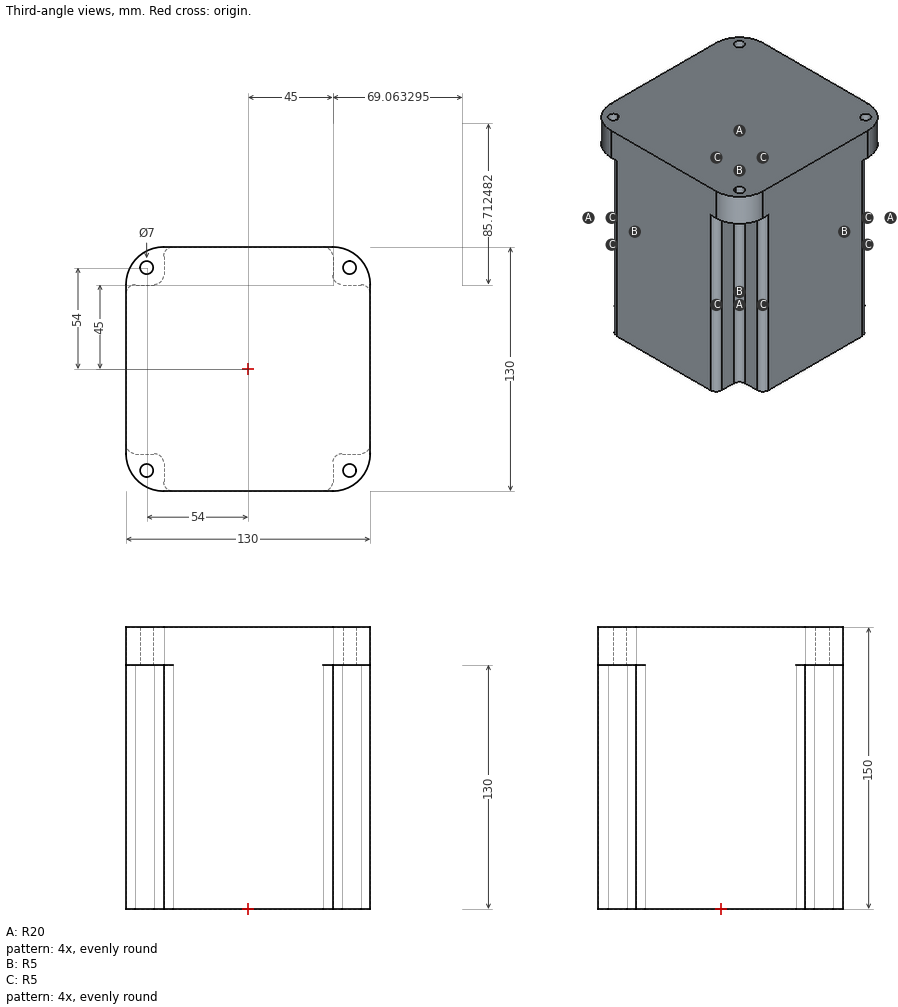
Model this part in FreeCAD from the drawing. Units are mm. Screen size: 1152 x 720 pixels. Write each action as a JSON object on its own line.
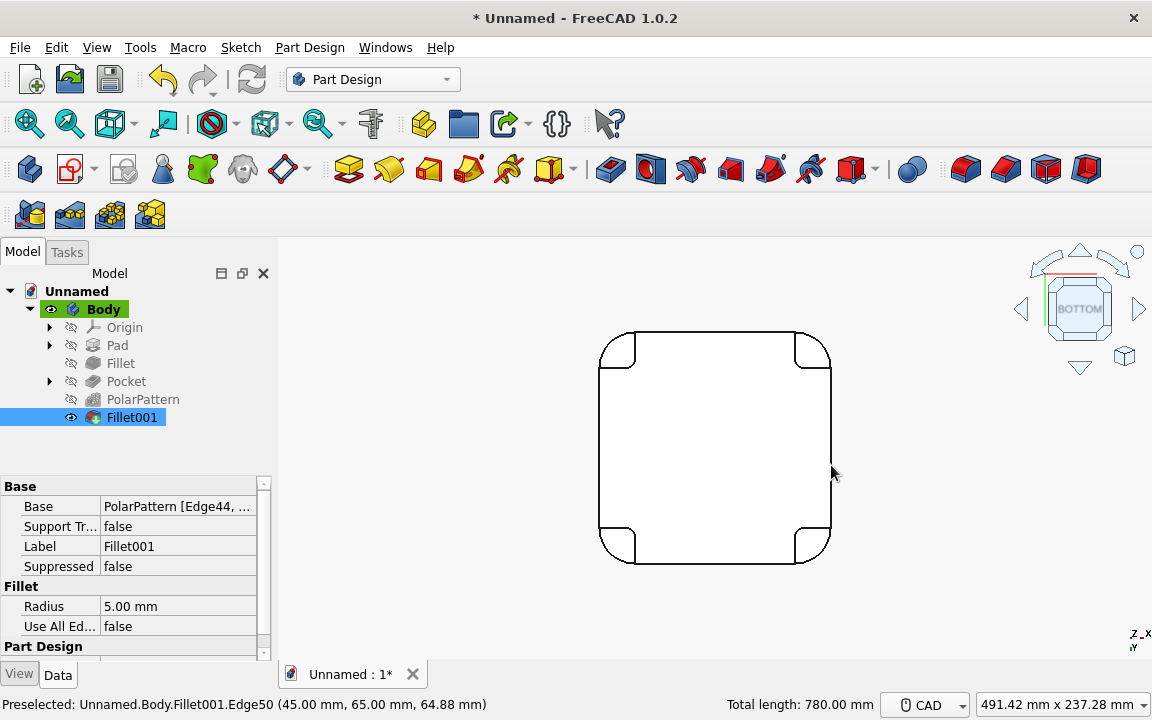
{"action": "key", "text": "4"}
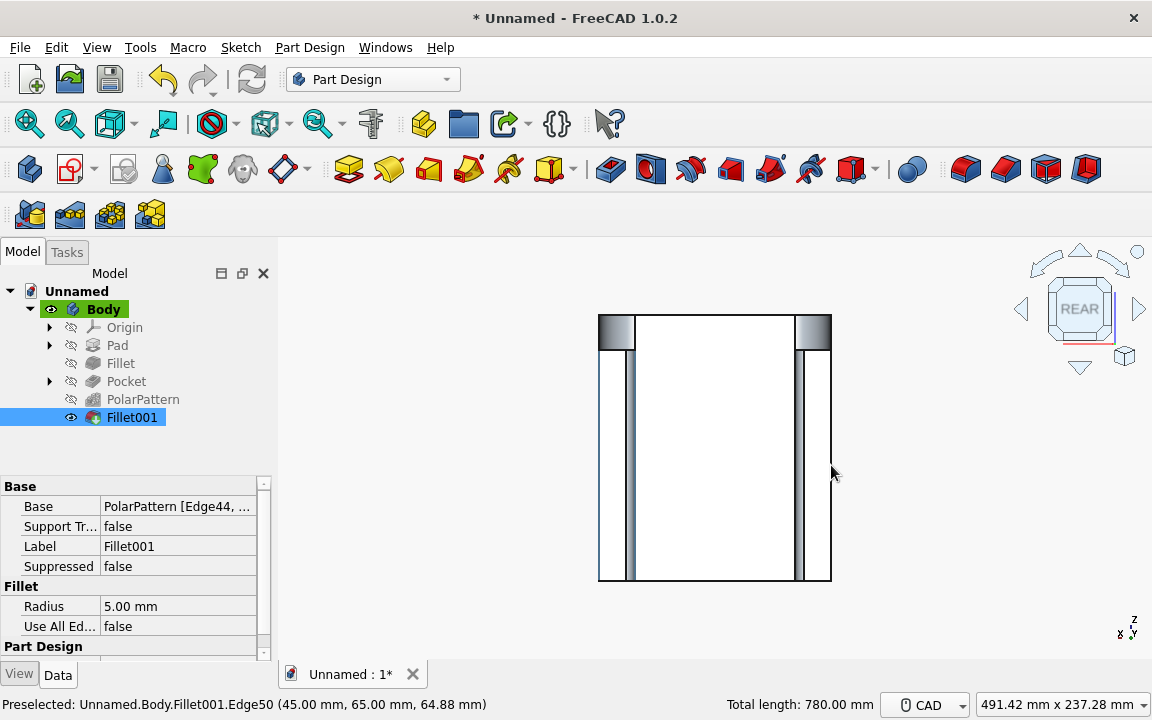
{"action": "left_click", "coordinate": [795, 465], "text": "ctrl"}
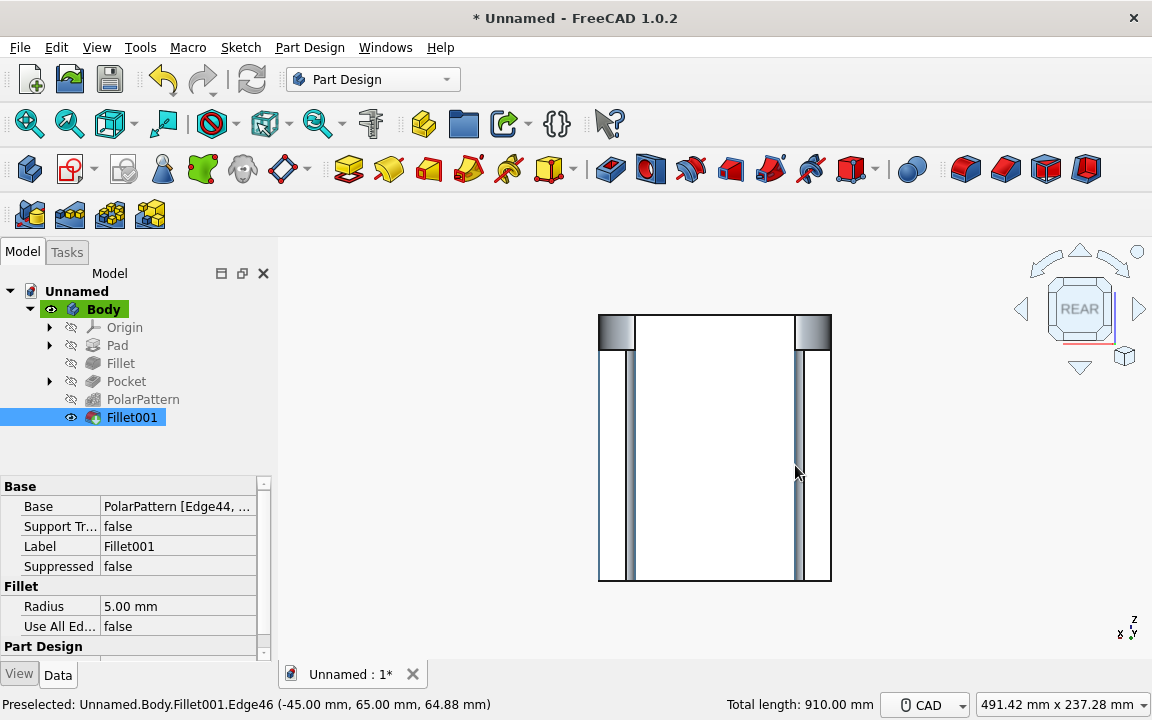
{"action": "left_click", "coordinate": [831, 465], "text": "ctrl"}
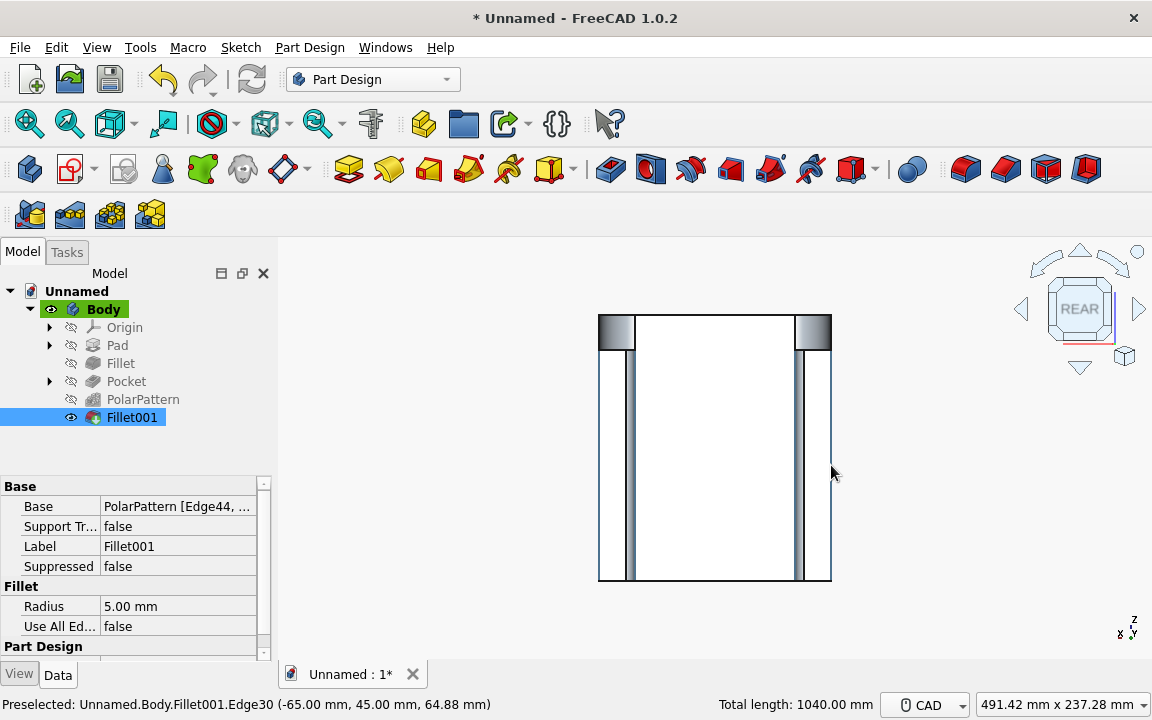
{"action": "left_click", "coordinate": [966, 170]}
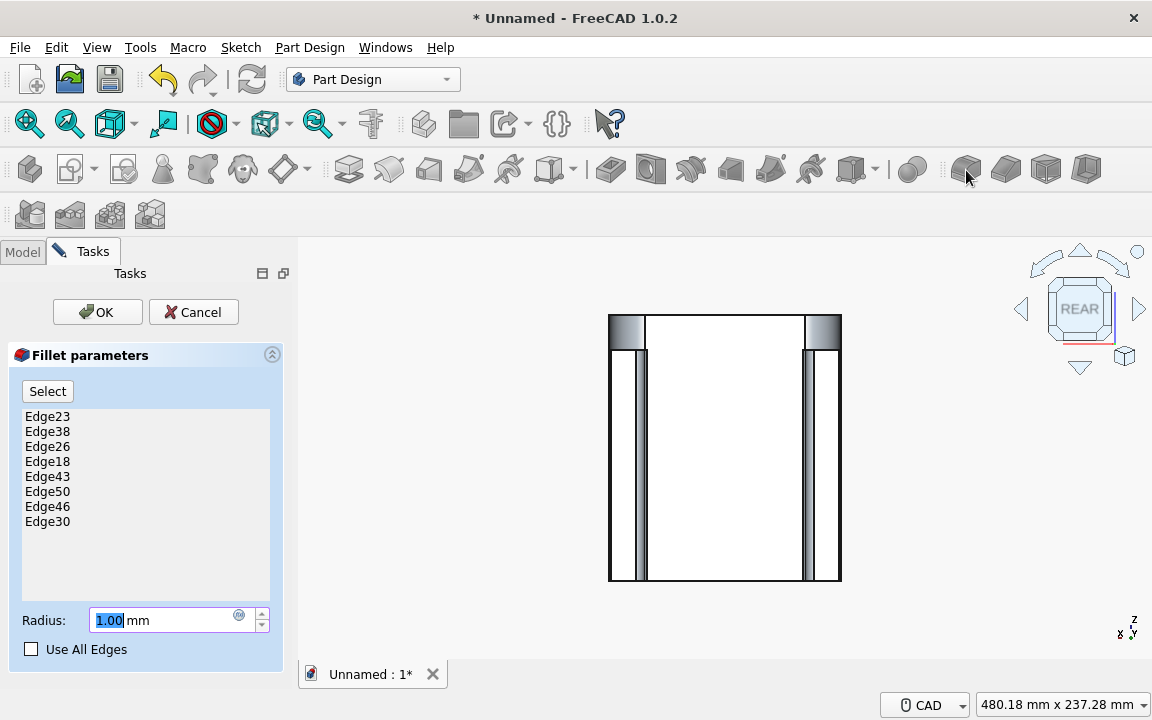
{"action": "type", "text": "5"}
{"action": "key", "text": "Tab"}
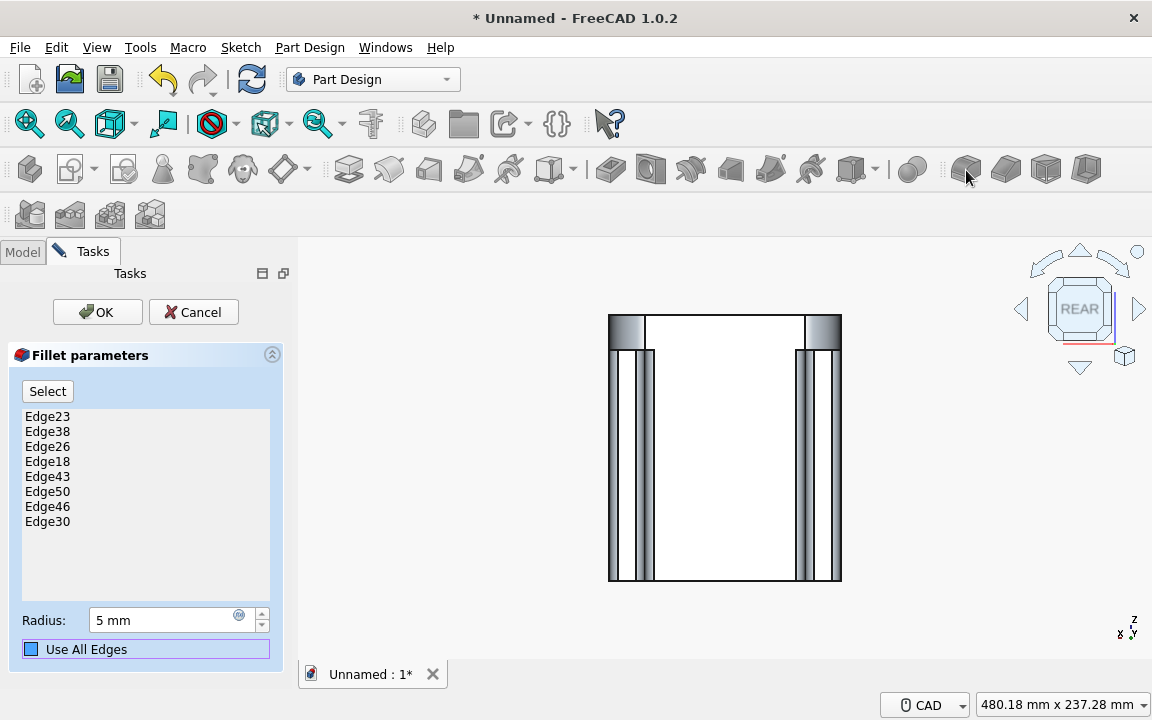
{"action": "left_click", "coordinate": [98, 312]}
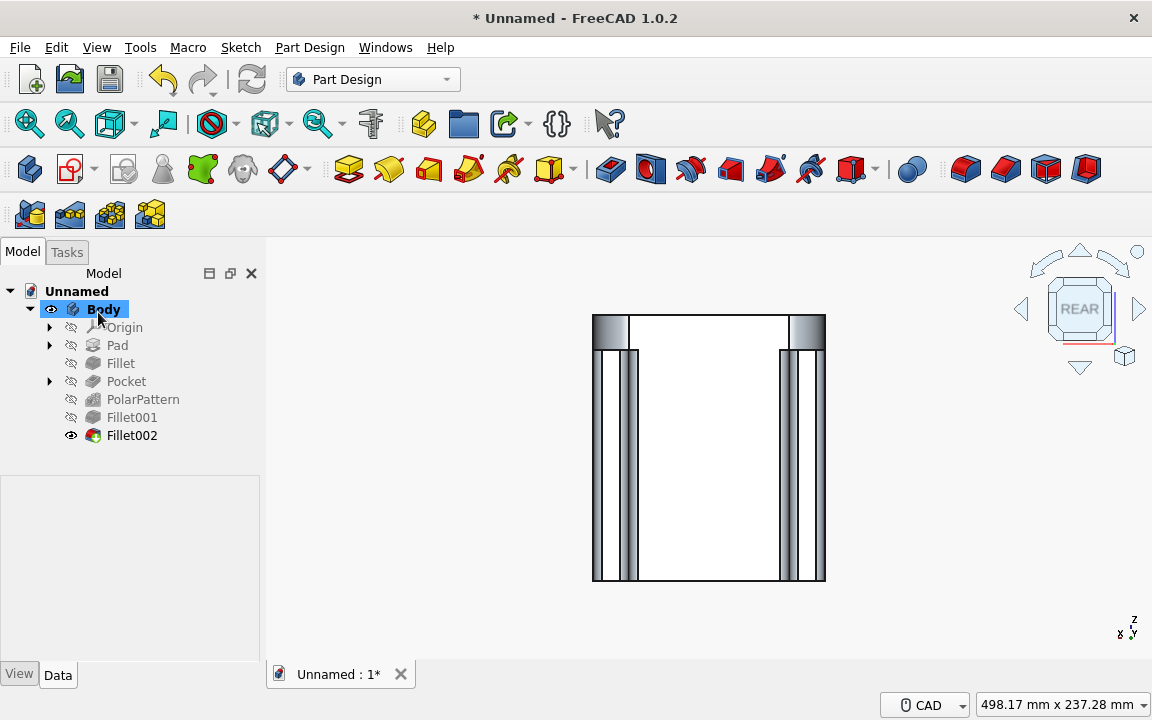
{"action": "key", "text": "5"}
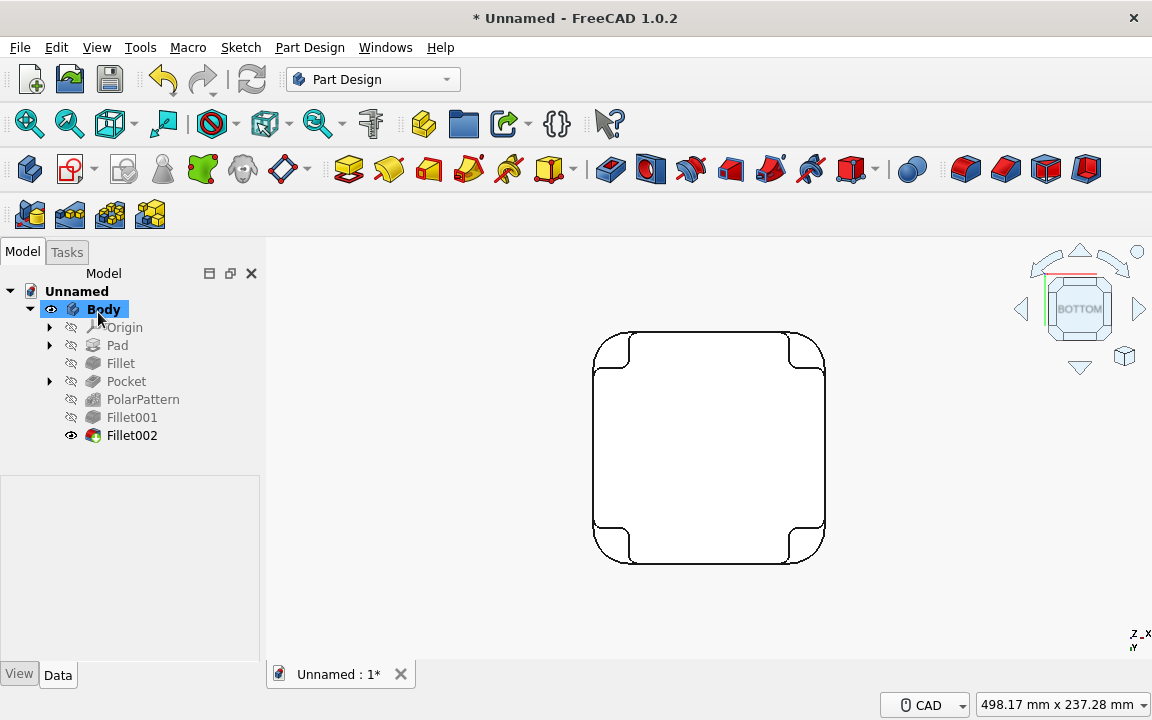
{"action": "left_click", "coordinate": [802, 354]}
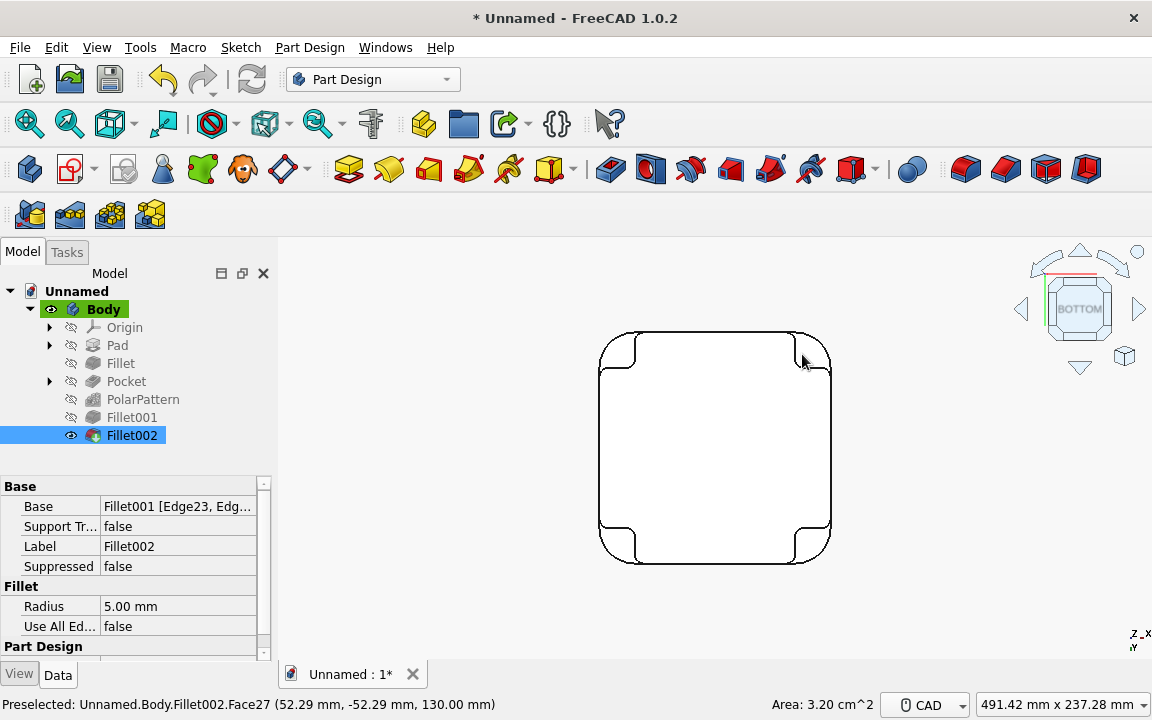
{"action": "left_click", "coordinate": [70, 170]}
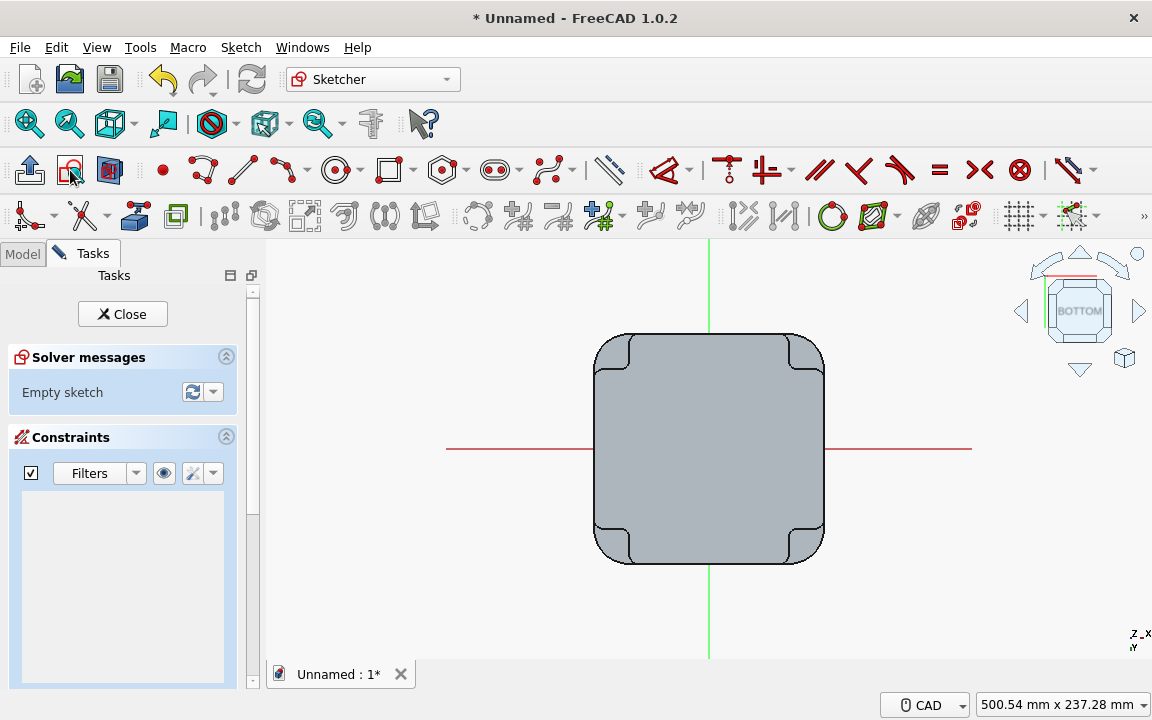
{"action": "scroll", "coordinate": [612, 550], "scroll_direction": "up", "scroll_amount": 15}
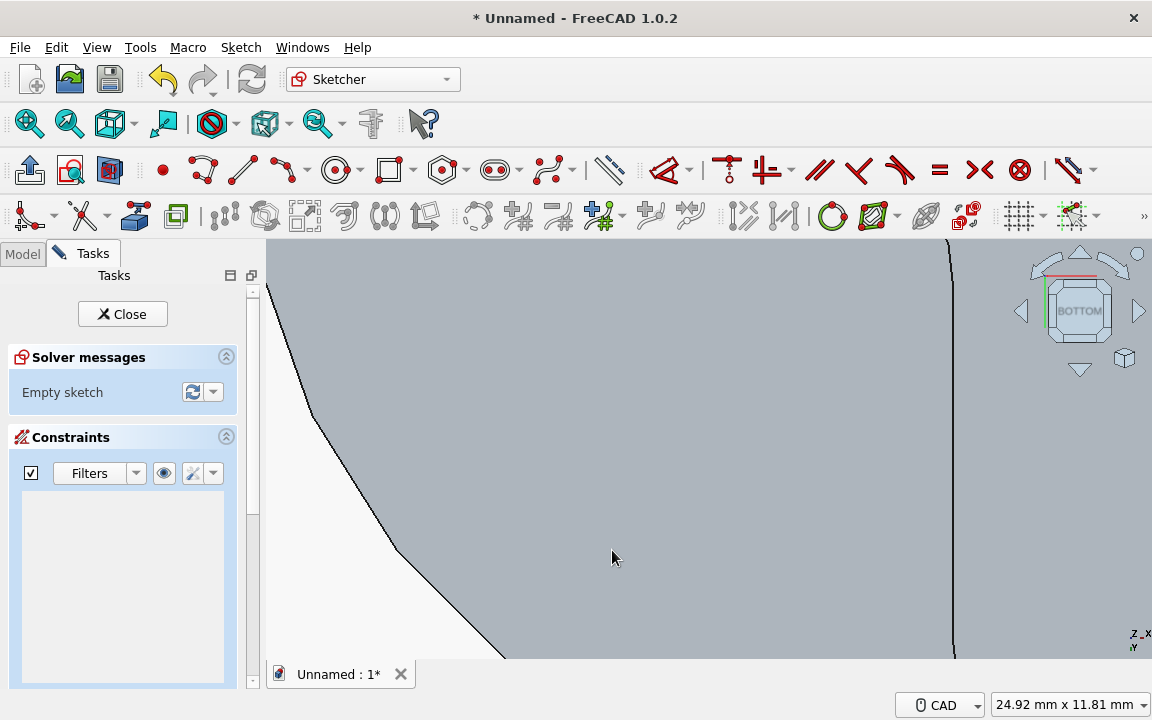
{"action": "left_click", "coordinate": [336, 170]}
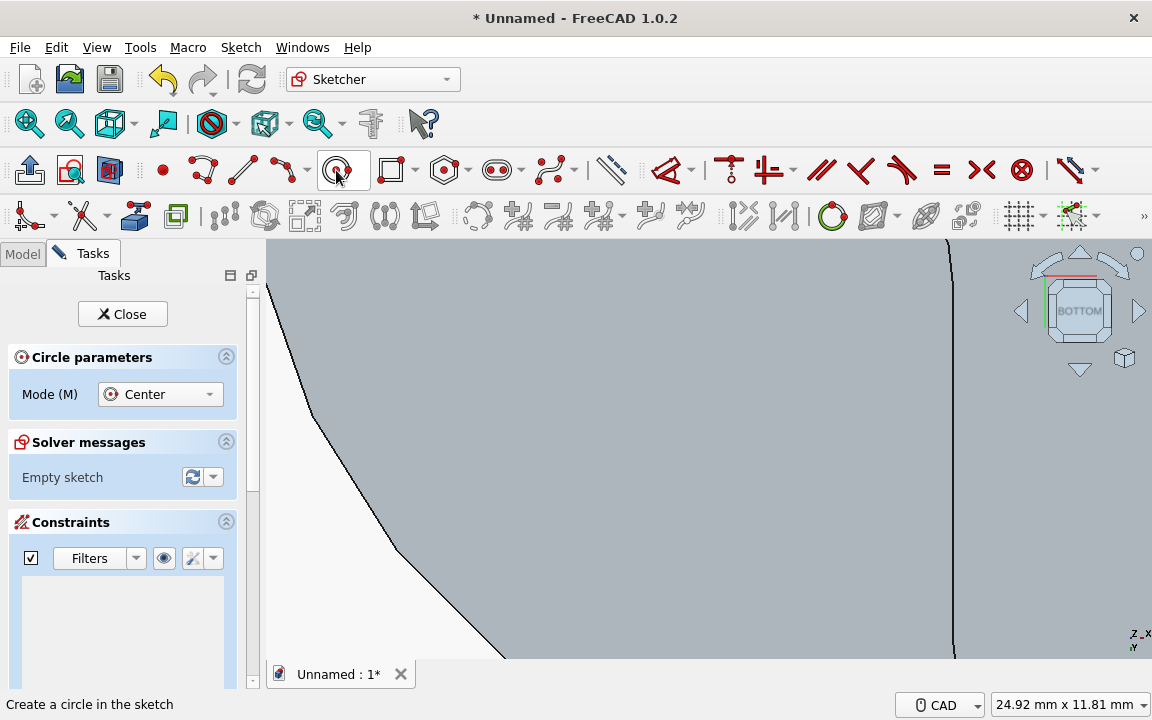
{"action": "left_click", "coordinate": [633, 427]}
{"action": "mouse_move", "coordinate": [721, 339]}